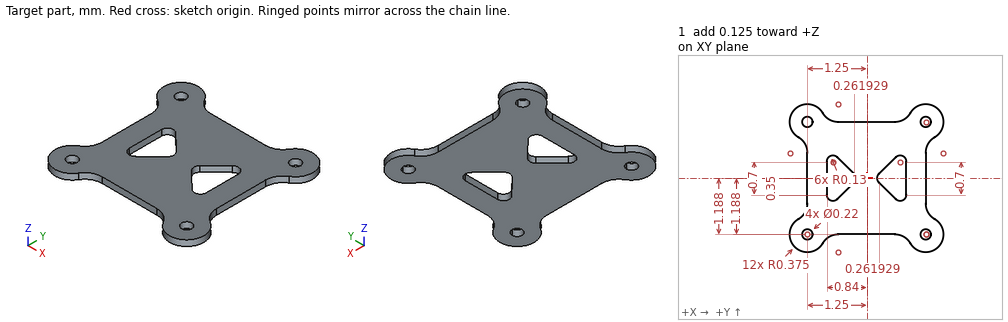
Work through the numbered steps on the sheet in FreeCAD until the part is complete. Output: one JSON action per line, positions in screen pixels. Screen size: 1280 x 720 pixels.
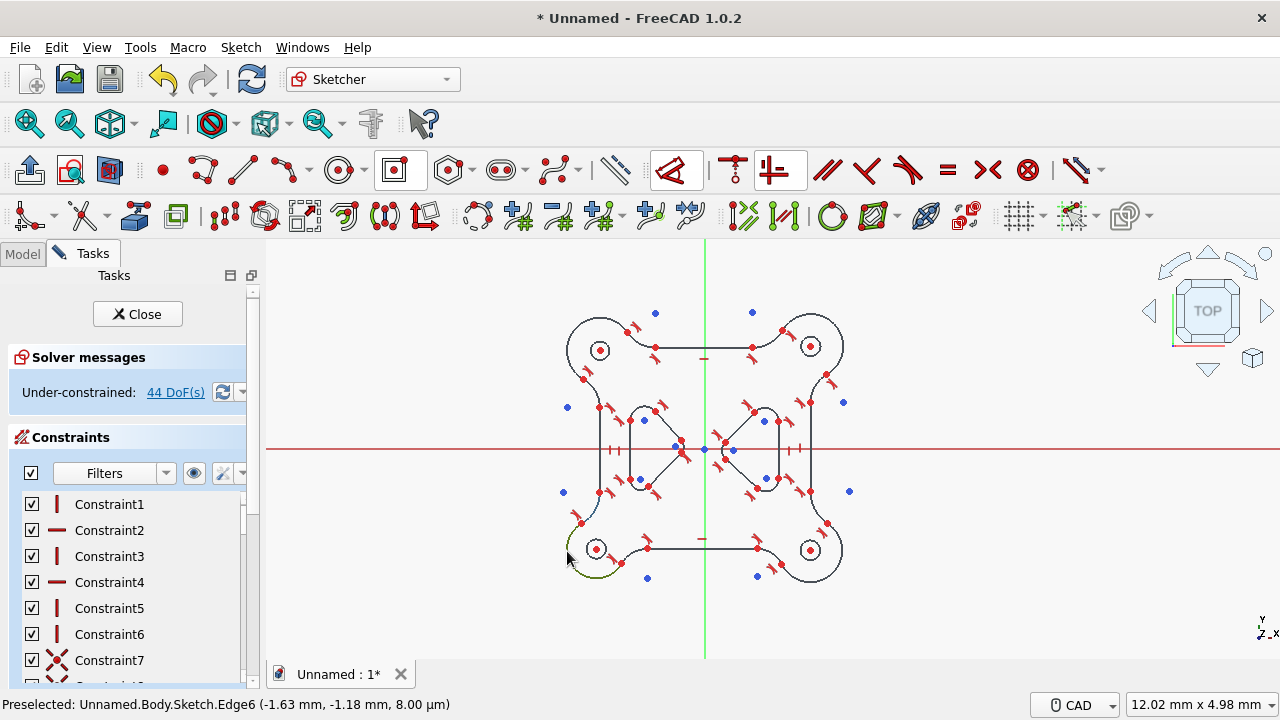
{"action": "scroll", "coordinate": [638, 550], "scroll_direction": "up", "scroll_amount": 3}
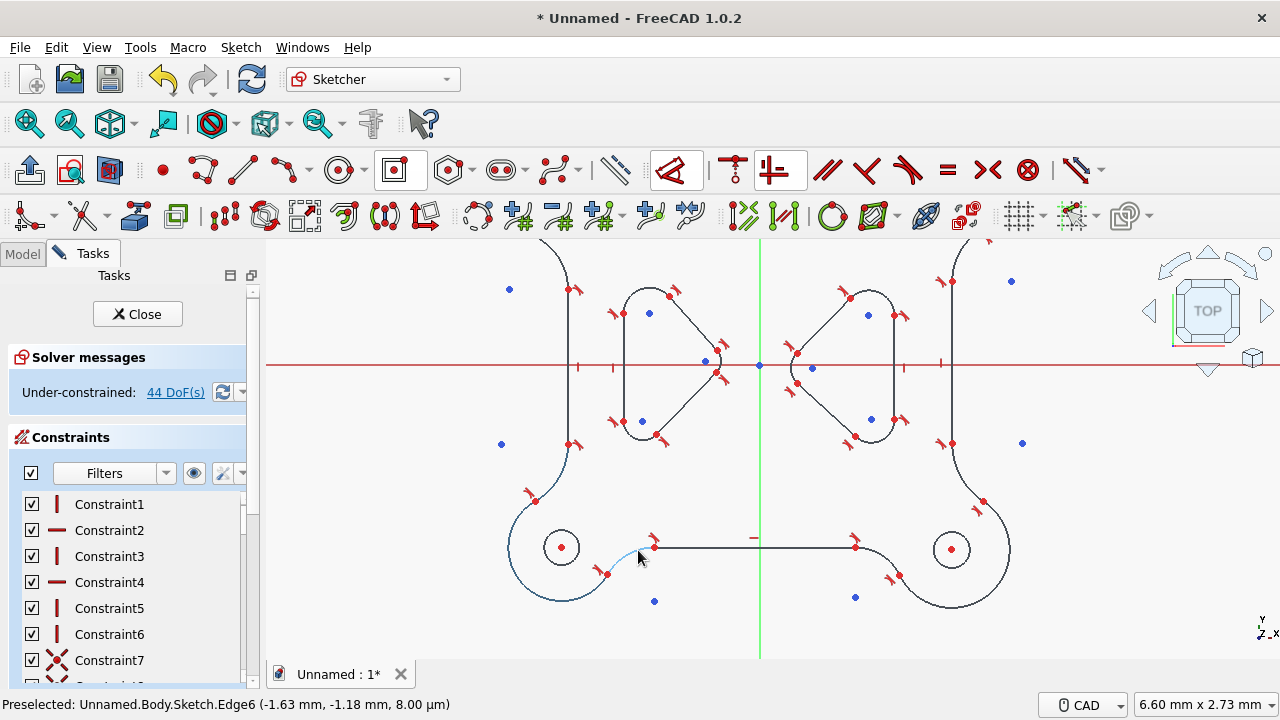
{"action": "left_click", "coordinate": [638, 550]}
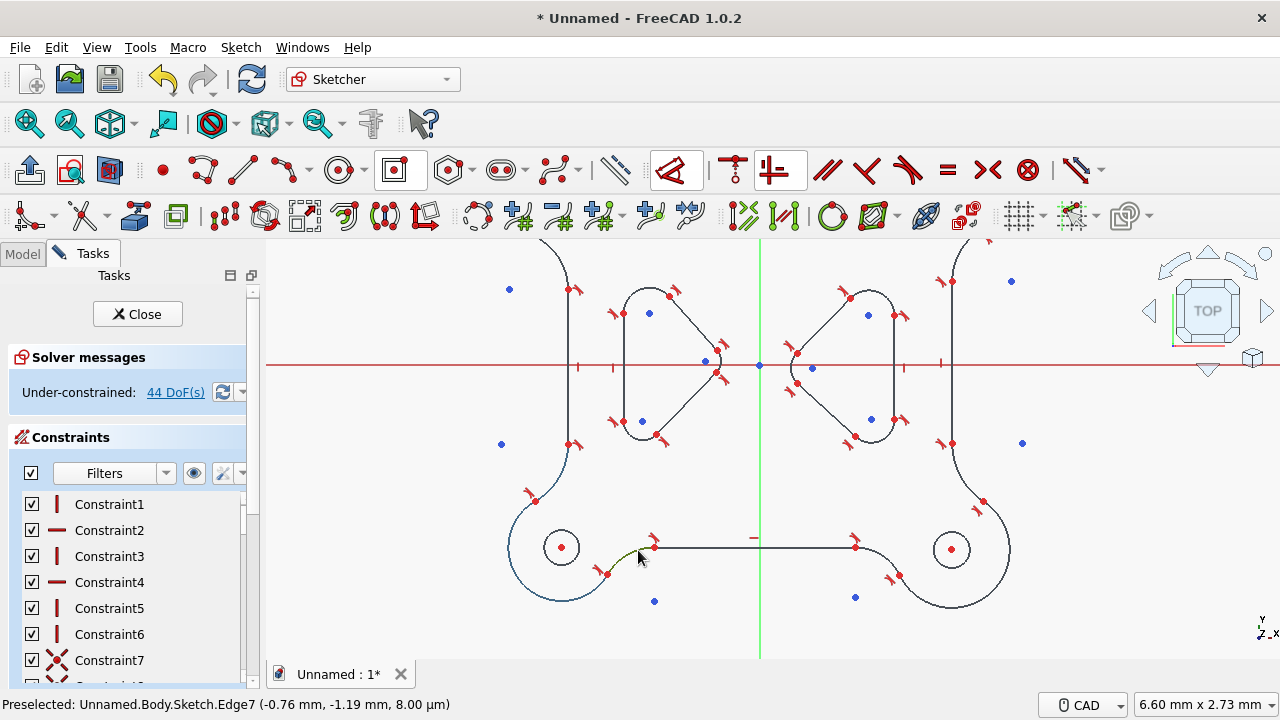
{"action": "left_click", "coordinate": [890, 562]}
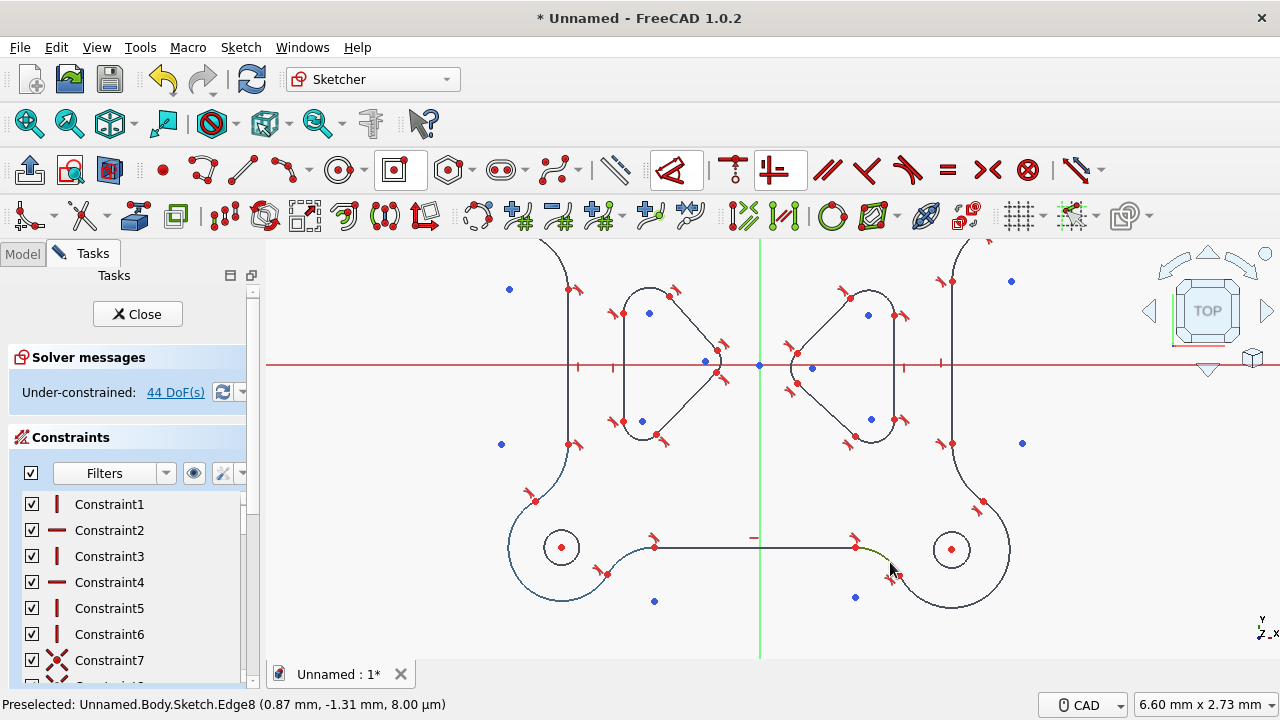
{"action": "left_click", "coordinate": [951, 608]}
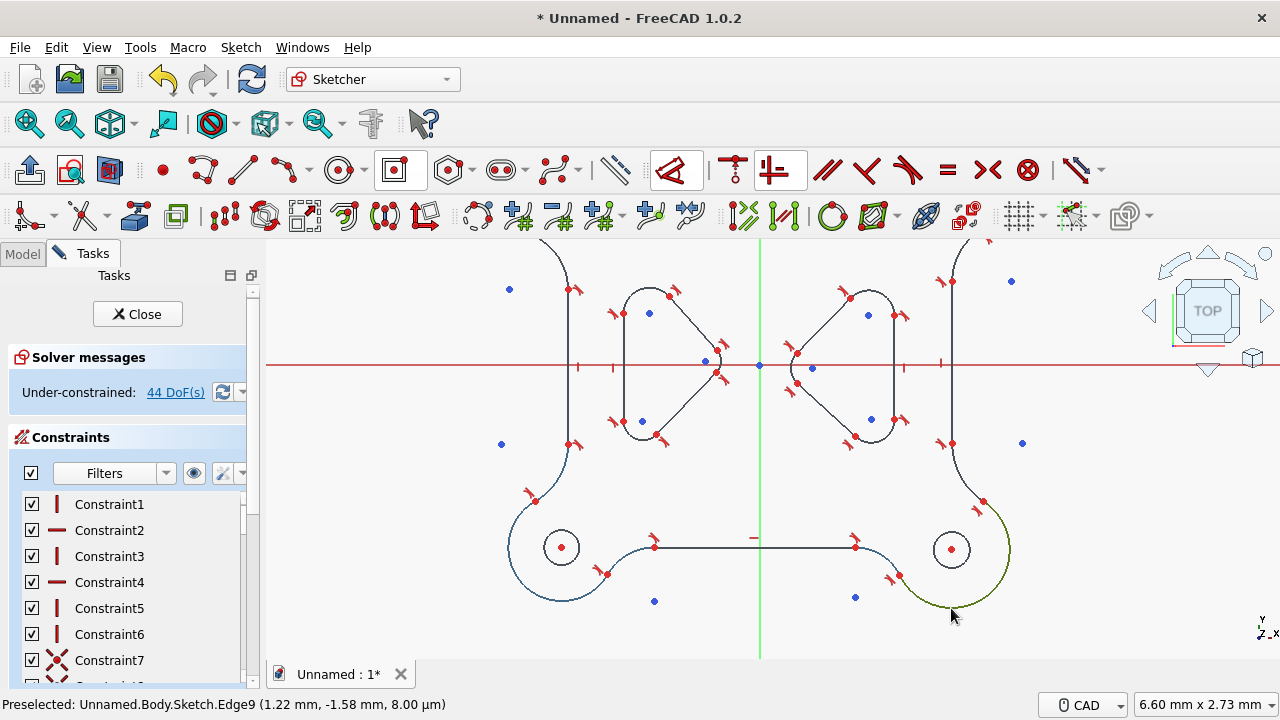
{"action": "left_click", "coordinate": [955, 464]}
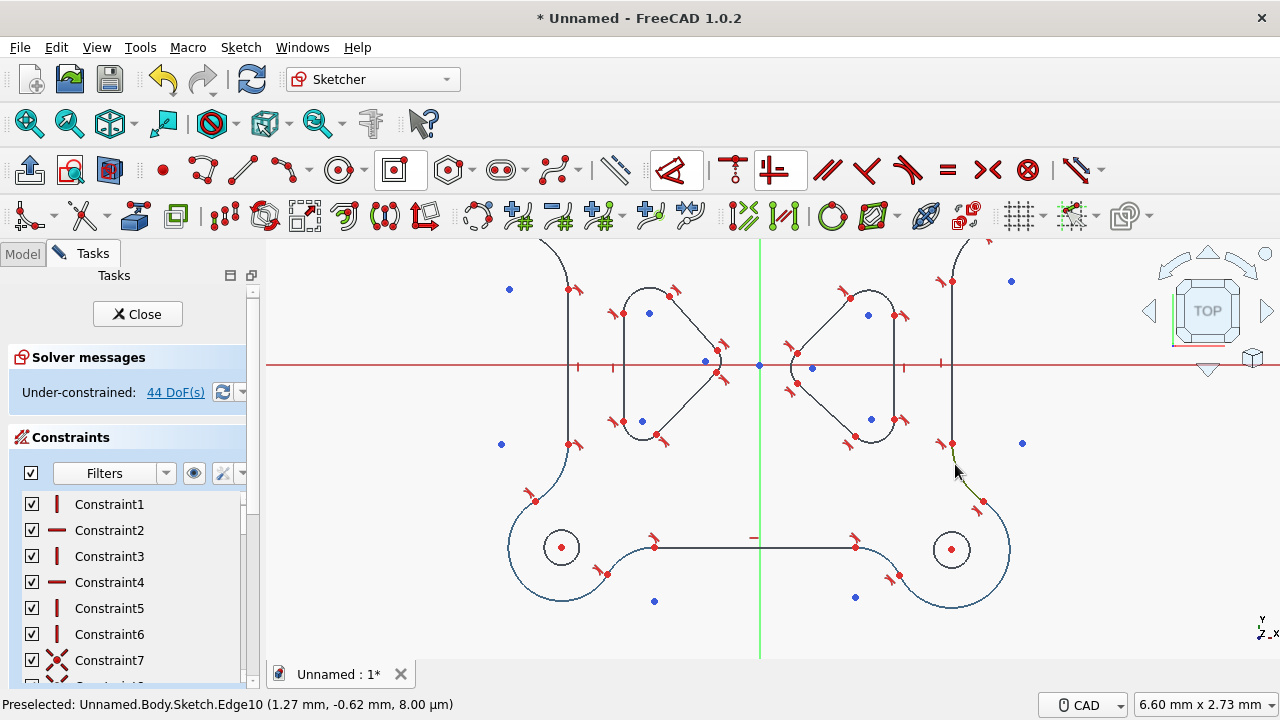
{"action": "left_click", "coordinate": [954, 269]}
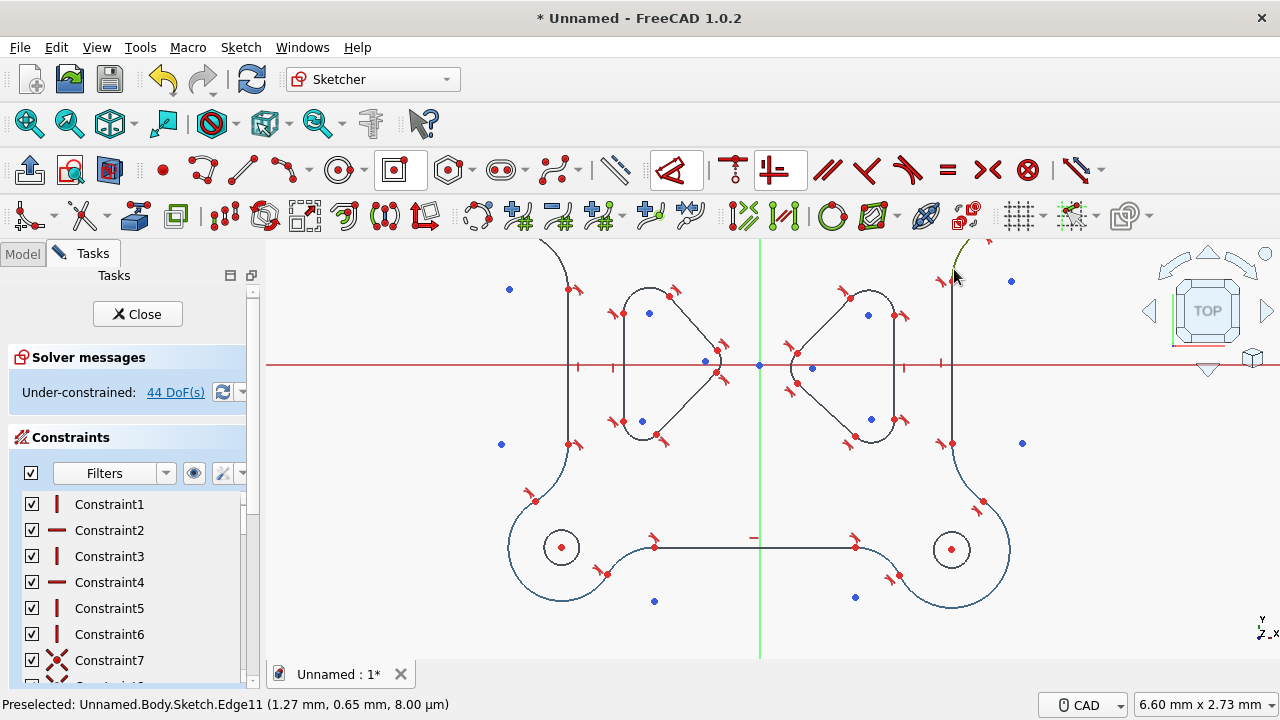
{"action": "scroll", "coordinate": [637, 551], "scroll_direction": "down", "scroll_amount": 3}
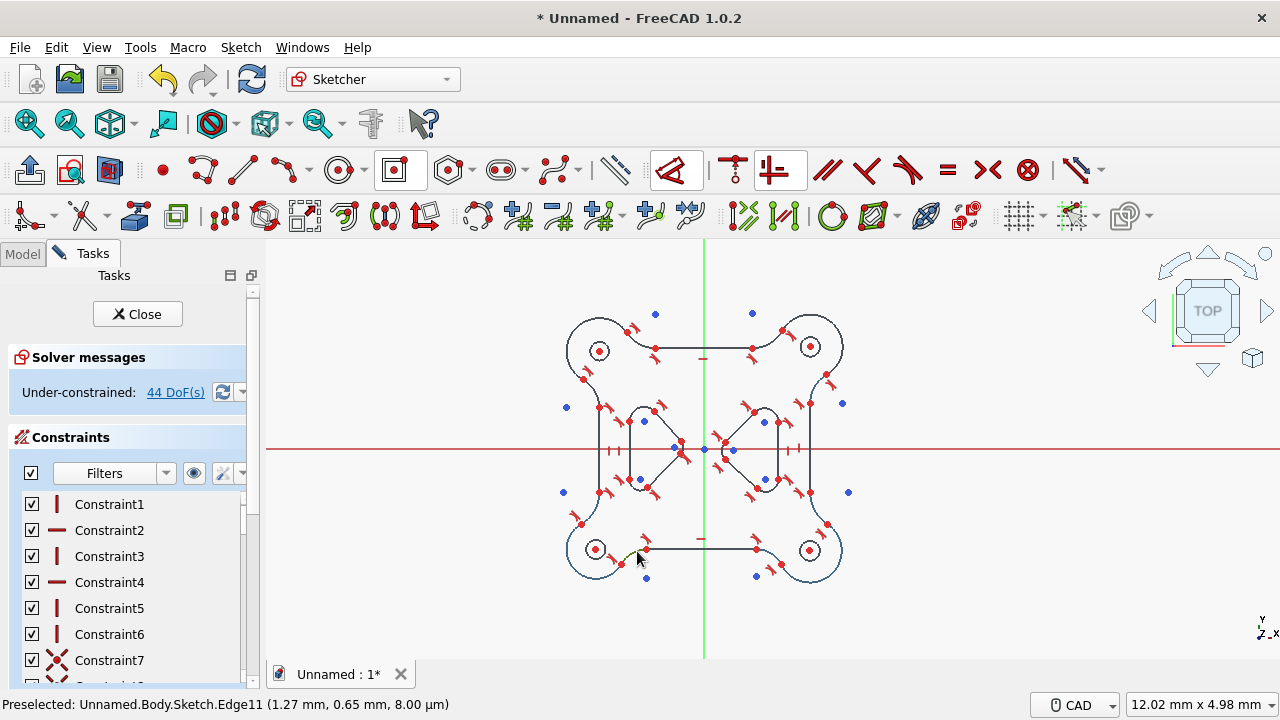
{"action": "left_click", "coordinate": [843, 345]}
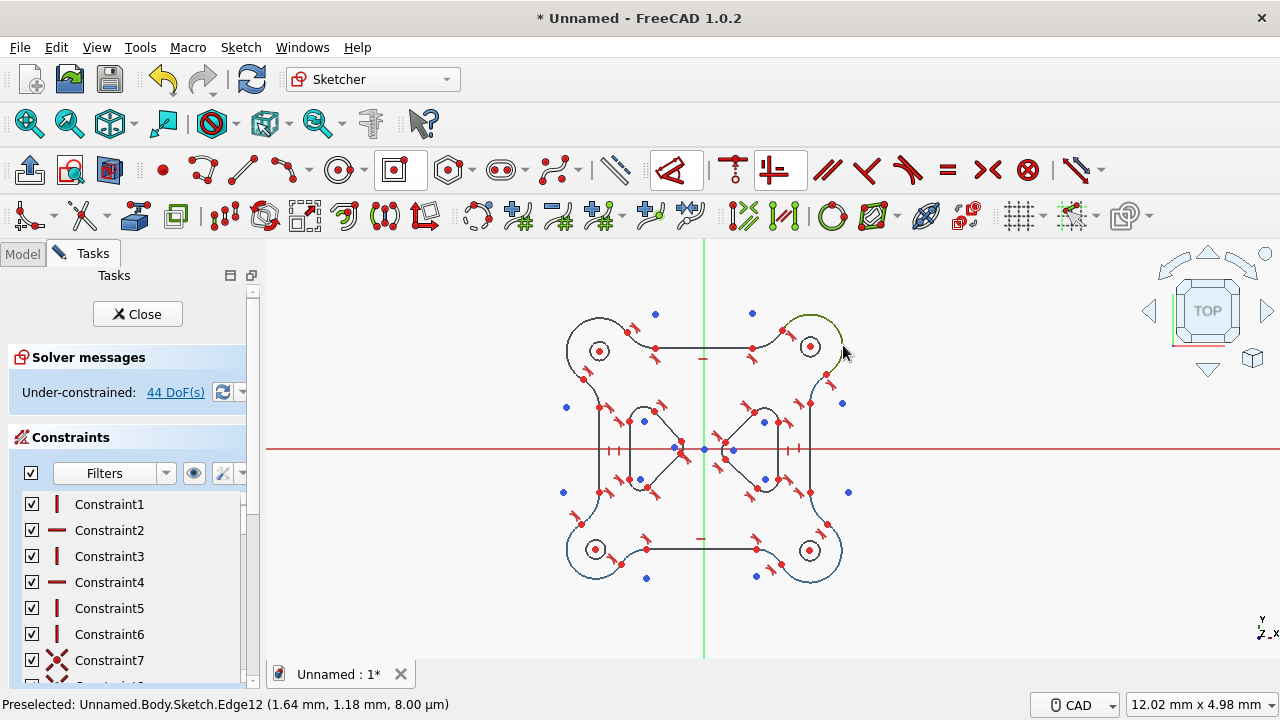
{"action": "scroll", "coordinate": [763, 346], "scroll_direction": "up", "scroll_amount": 2}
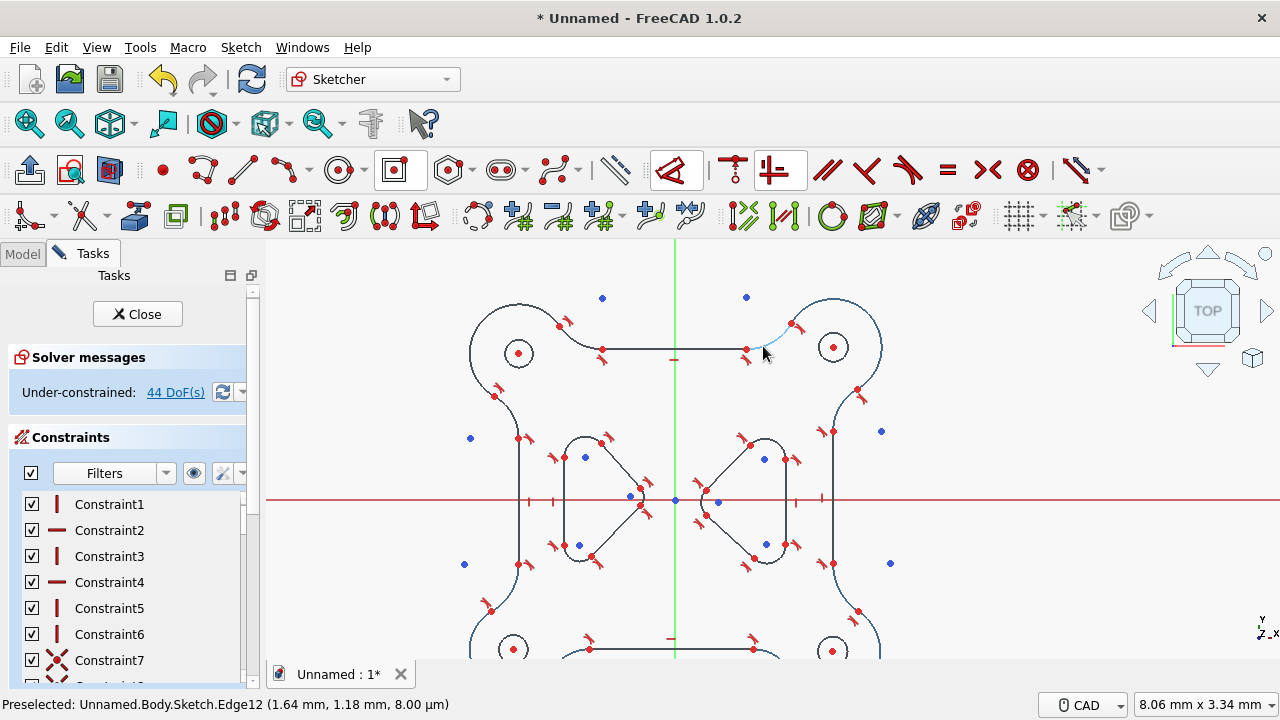
{"action": "left_click", "coordinate": [763, 347]}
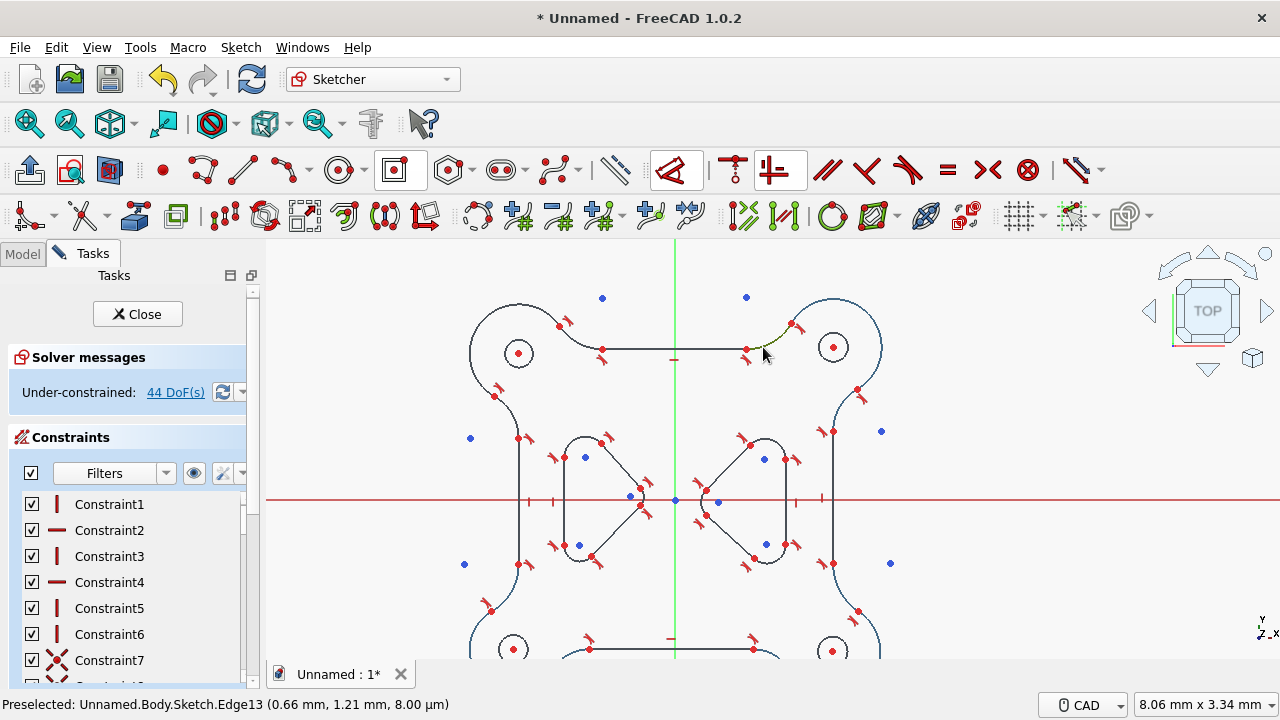
{"action": "left_click", "coordinate": [570, 338]}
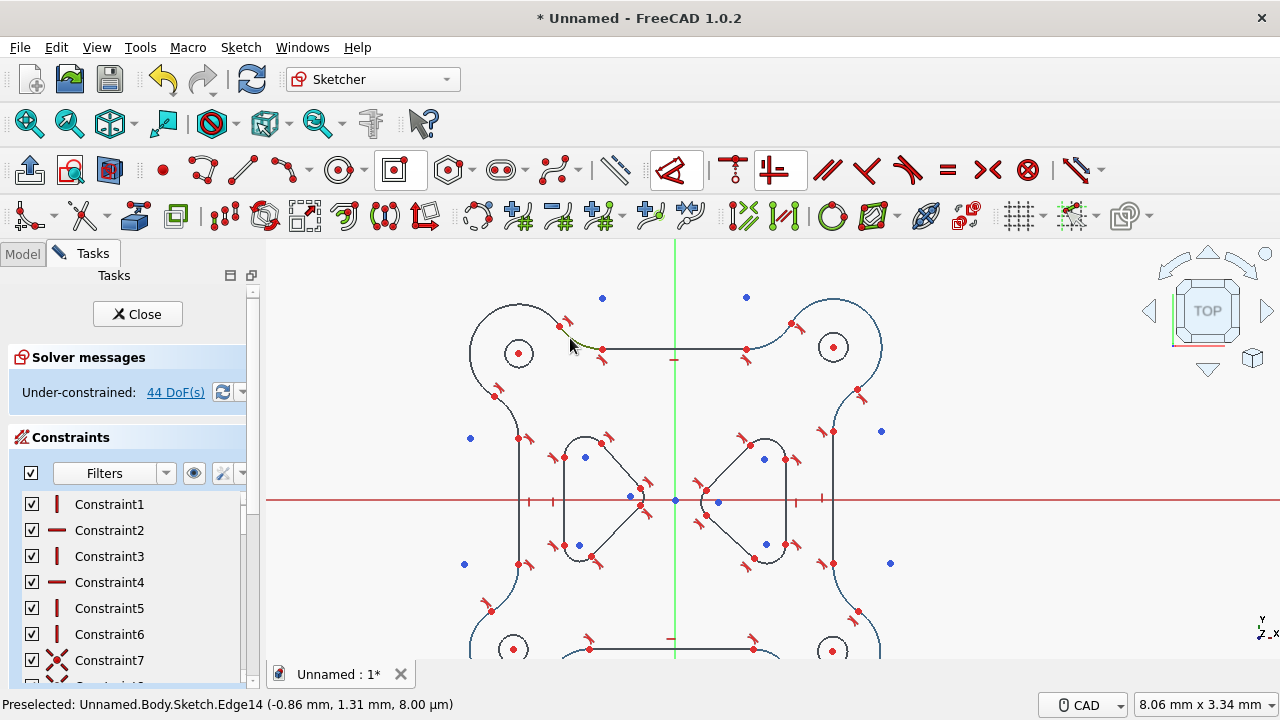
{"action": "left_click", "coordinate": [514, 305]}